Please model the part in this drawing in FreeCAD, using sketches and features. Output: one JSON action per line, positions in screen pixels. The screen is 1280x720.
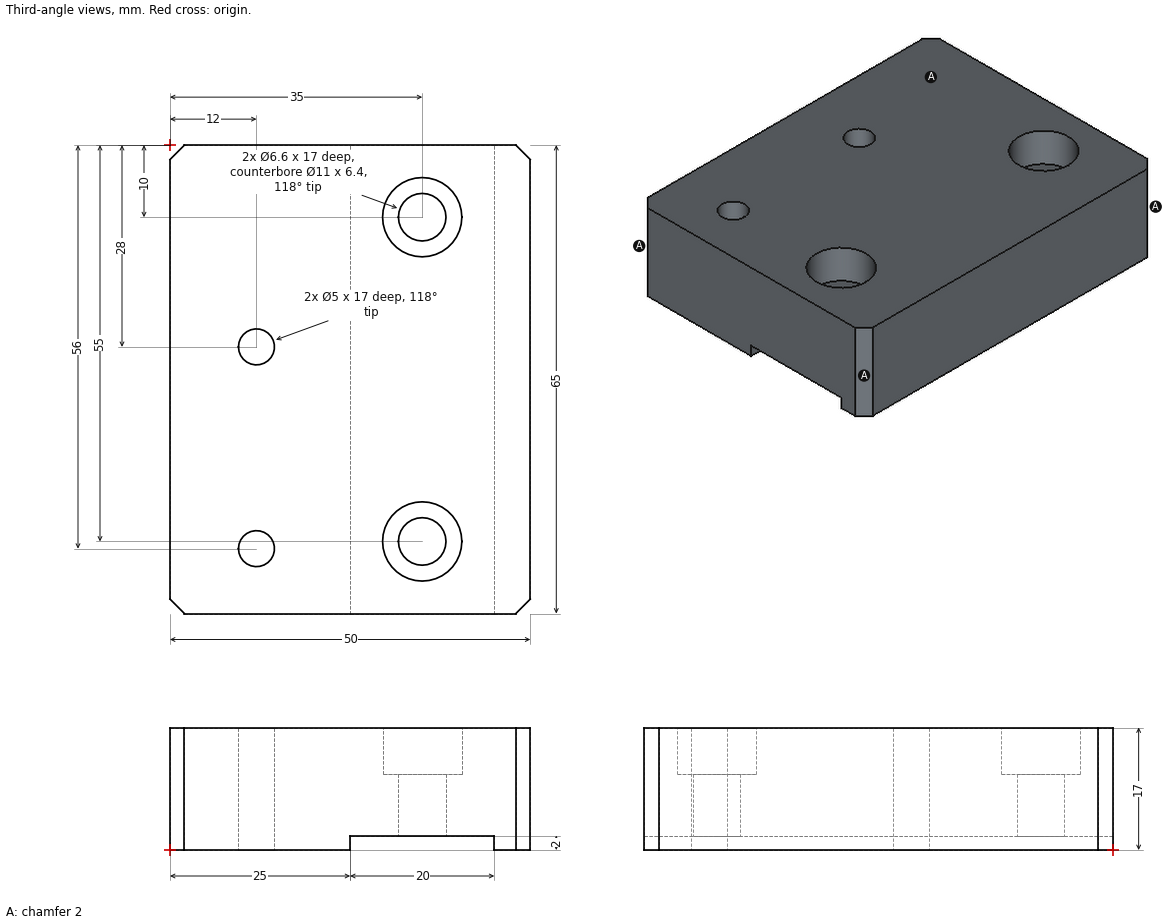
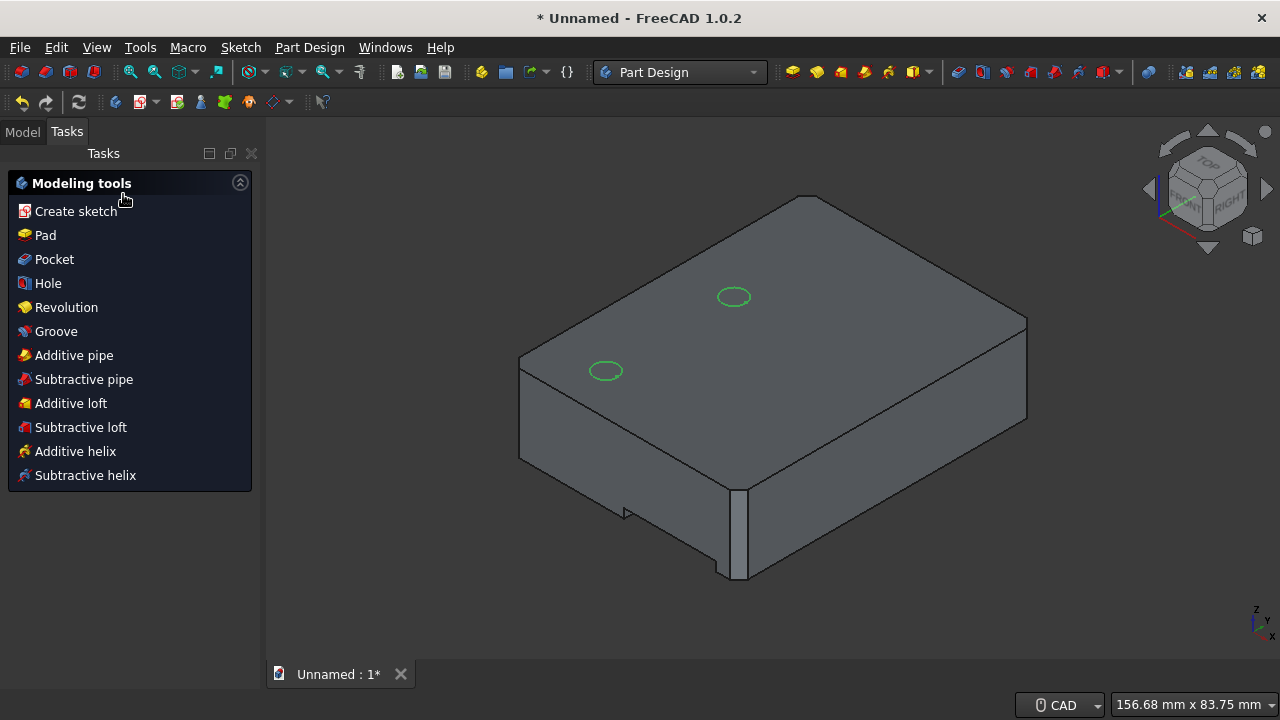
{"action": "left_click", "coordinate": [984, 72]}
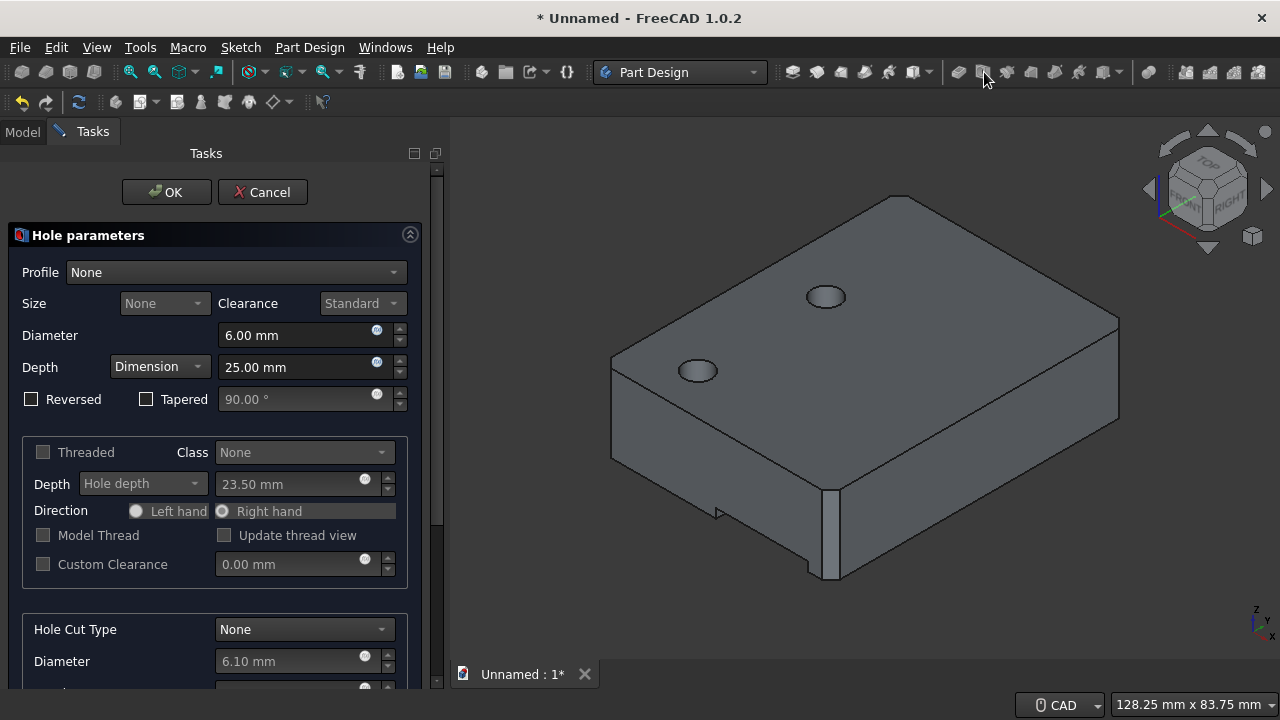
{"action": "triple_click", "coordinate": [305, 335]}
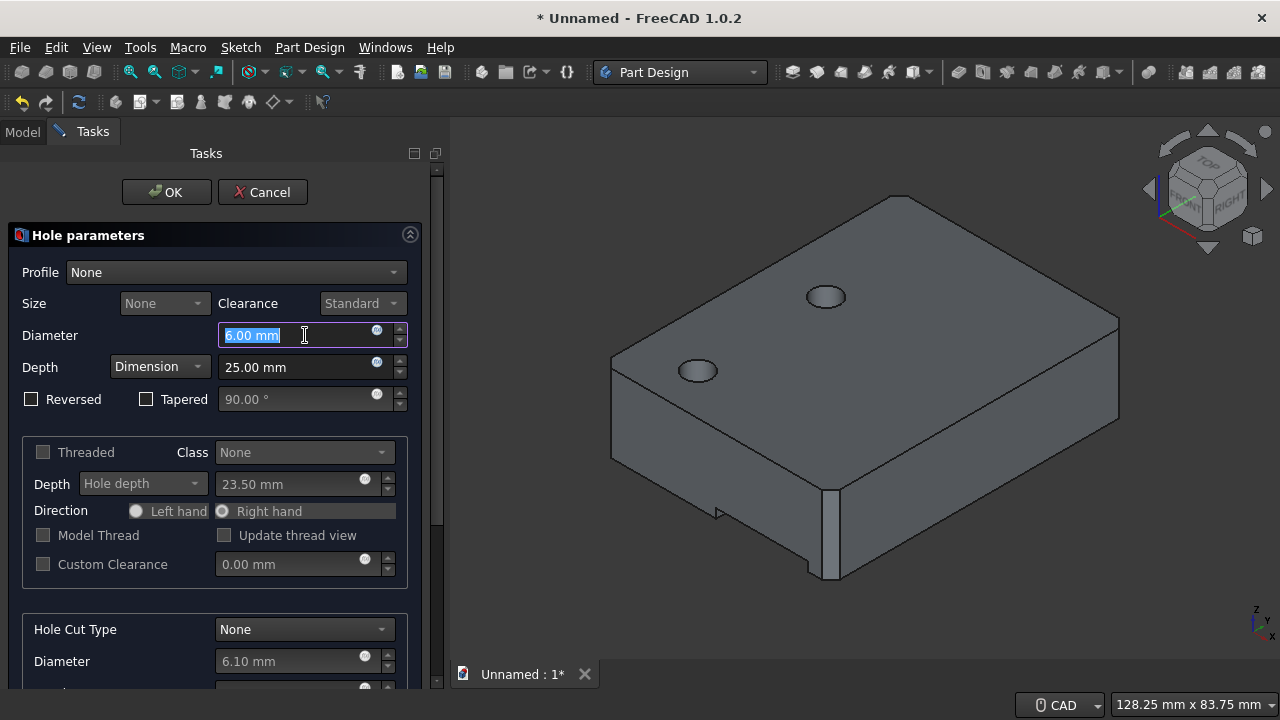
{"action": "type", "text": "5"}
{"action": "key", "text": "Tab"}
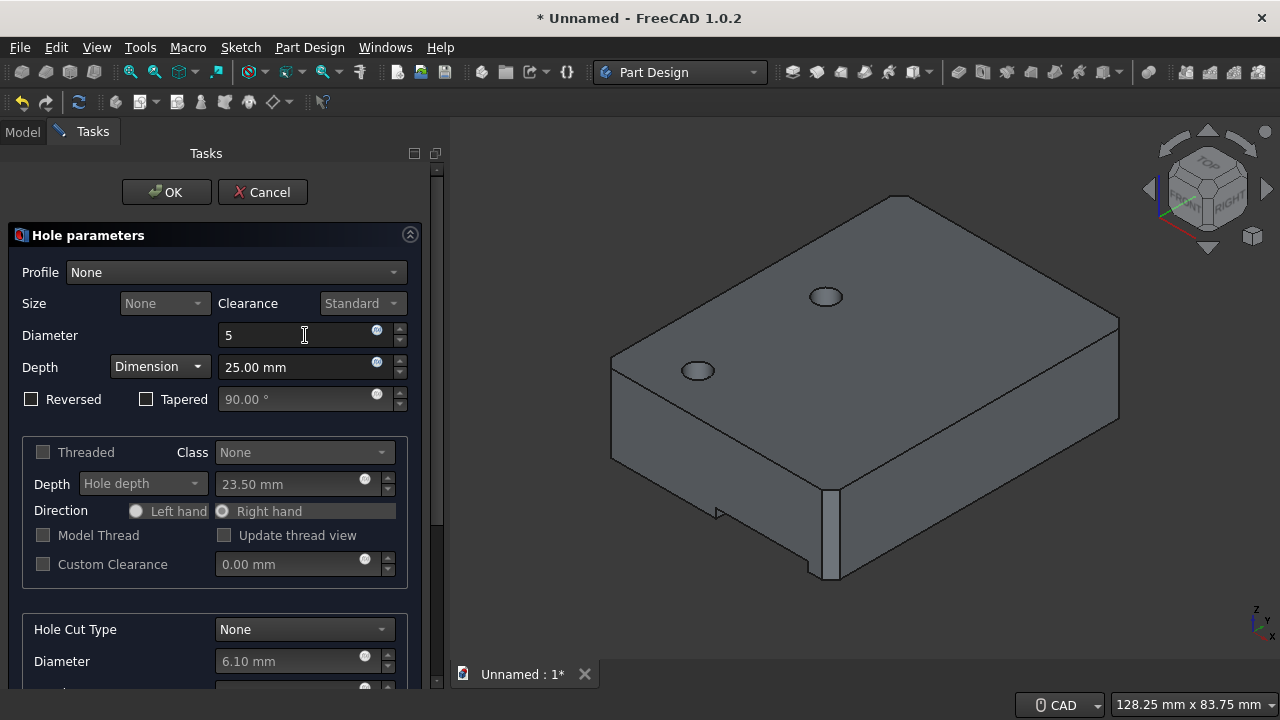
{"action": "triple_click", "coordinate": [305, 367]}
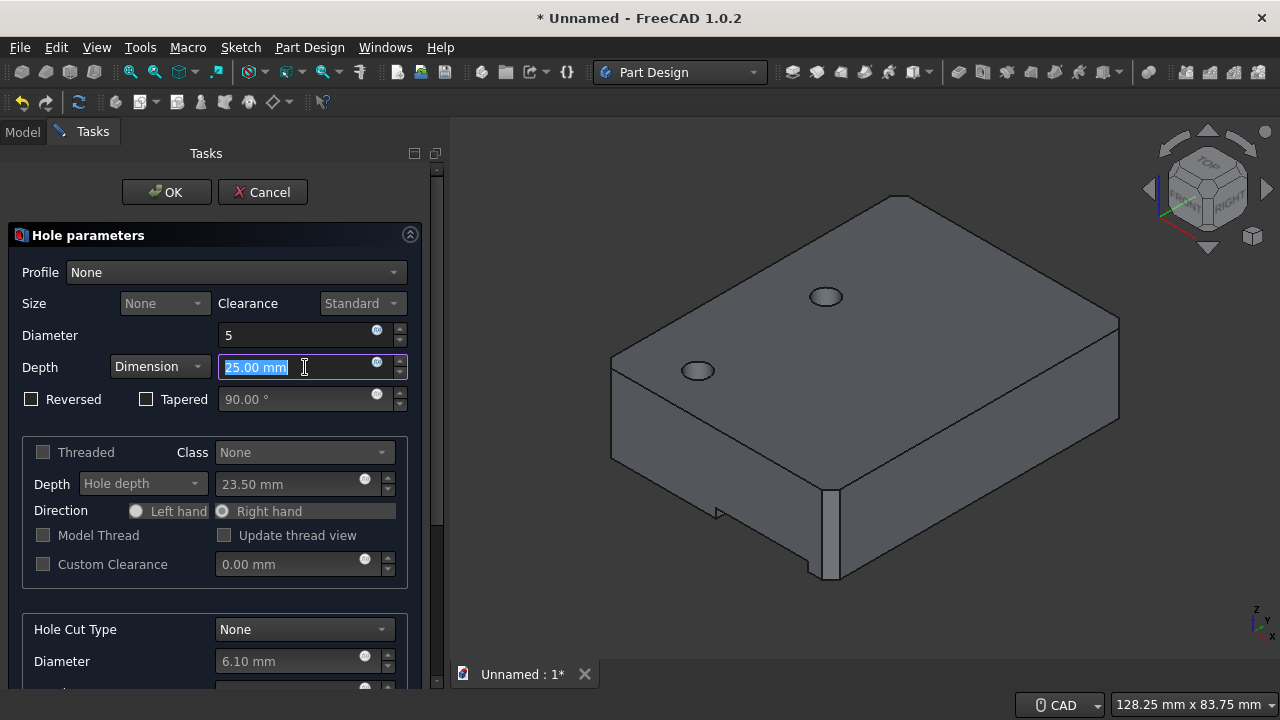
{"action": "type", "text": "17"}
{"action": "key", "text": "Tab"}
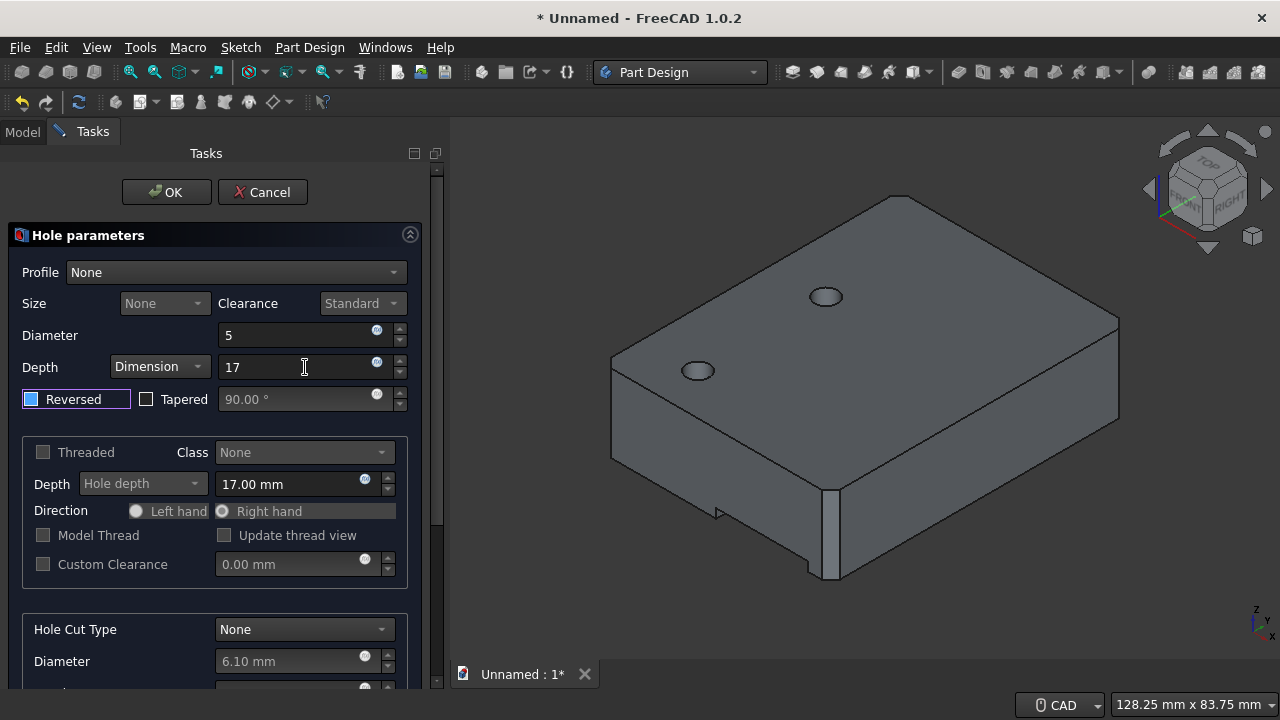
{"action": "left_click", "coordinate": [167, 192]}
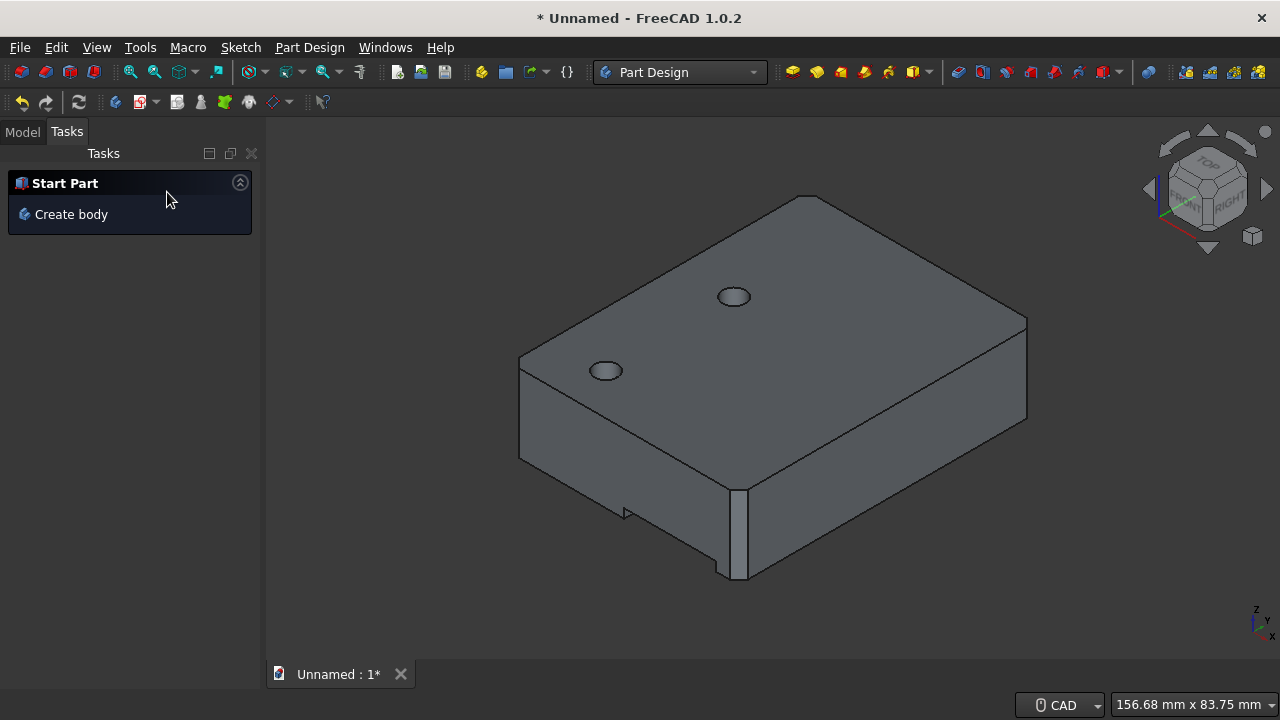
{"action": "left_click", "coordinate": [848, 336]}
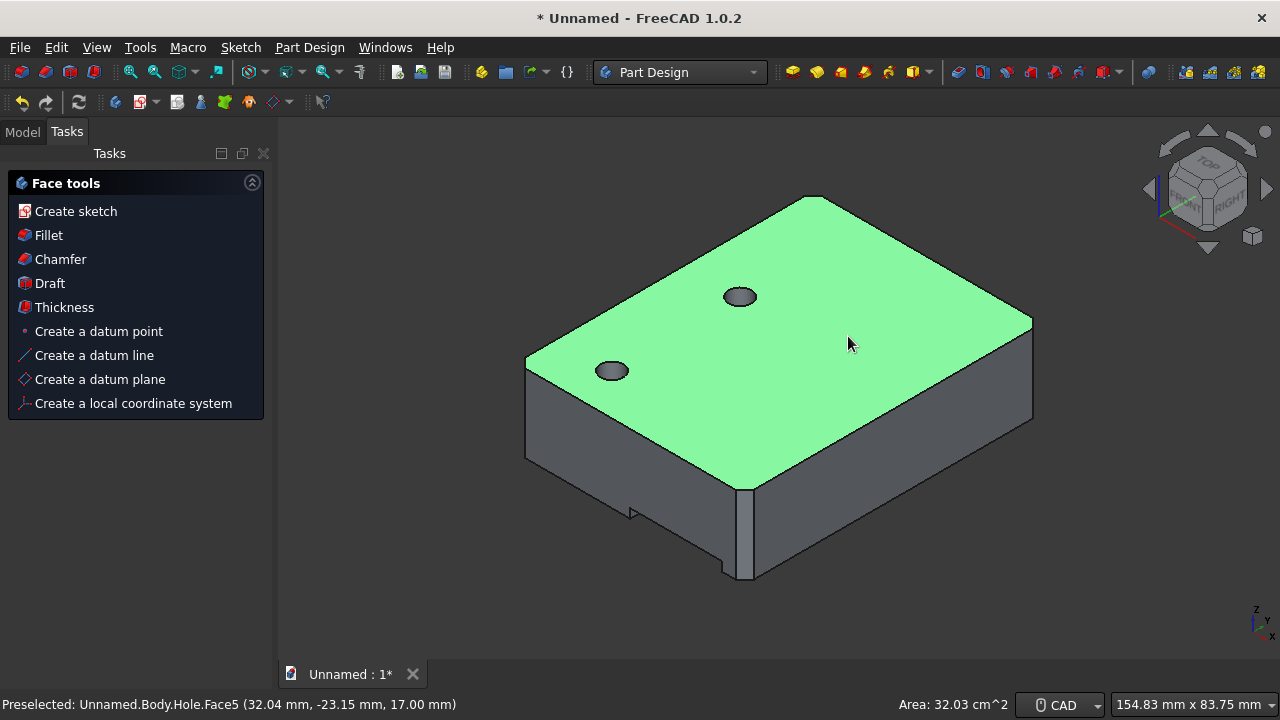
{"action": "left_click", "coordinate": [140, 102]}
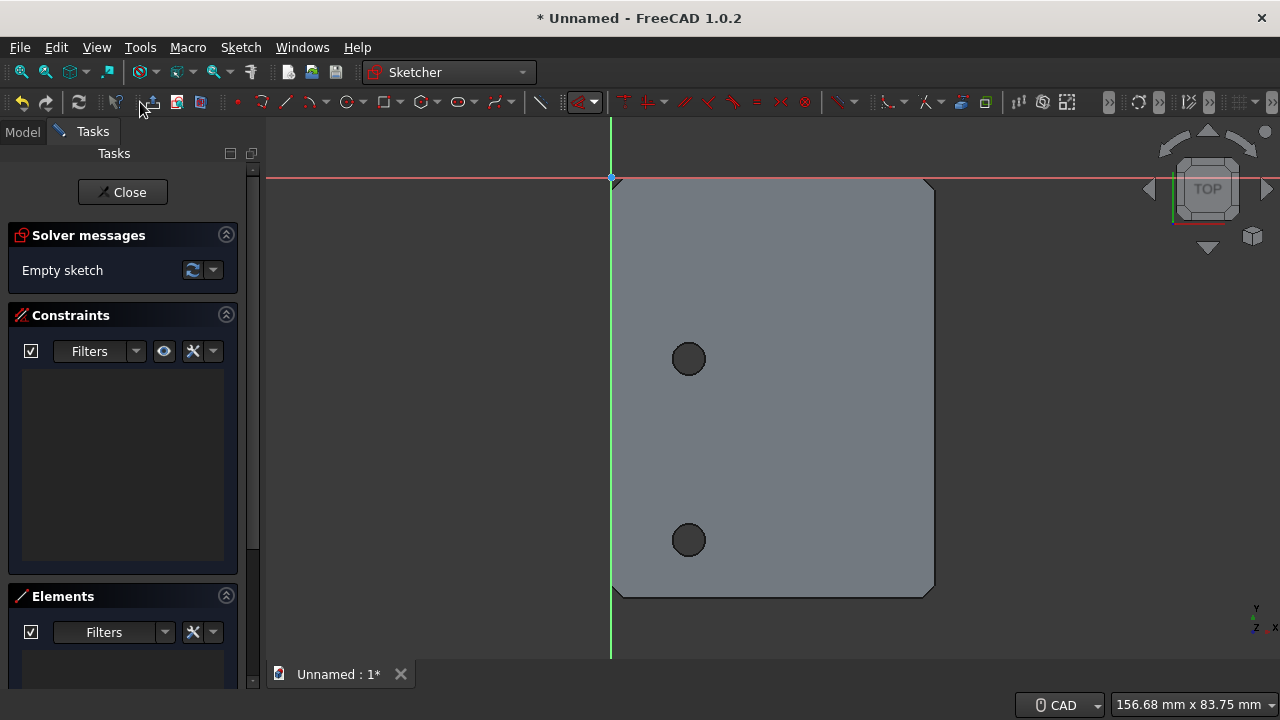
{"action": "left_click", "coordinate": [348, 102]}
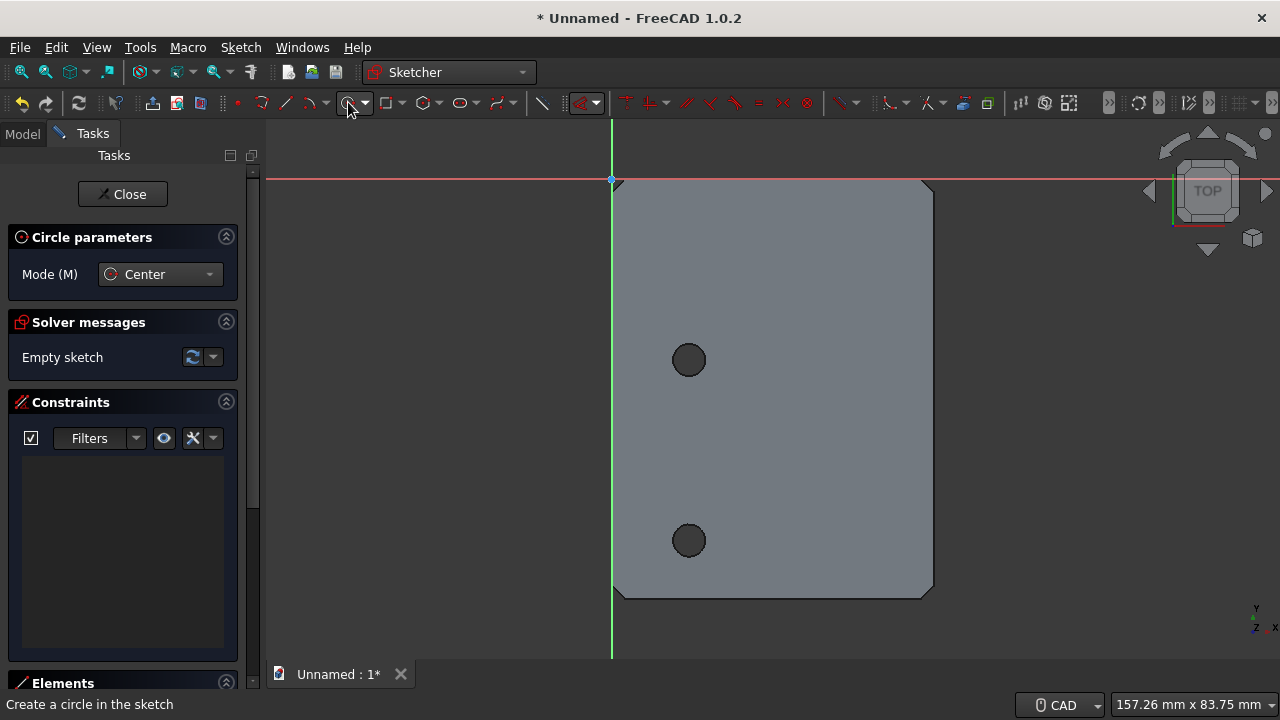
{"action": "left_click", "coordinate": [837, 244]}
{"action": "mouse_move", "coordinate": [853, 229]}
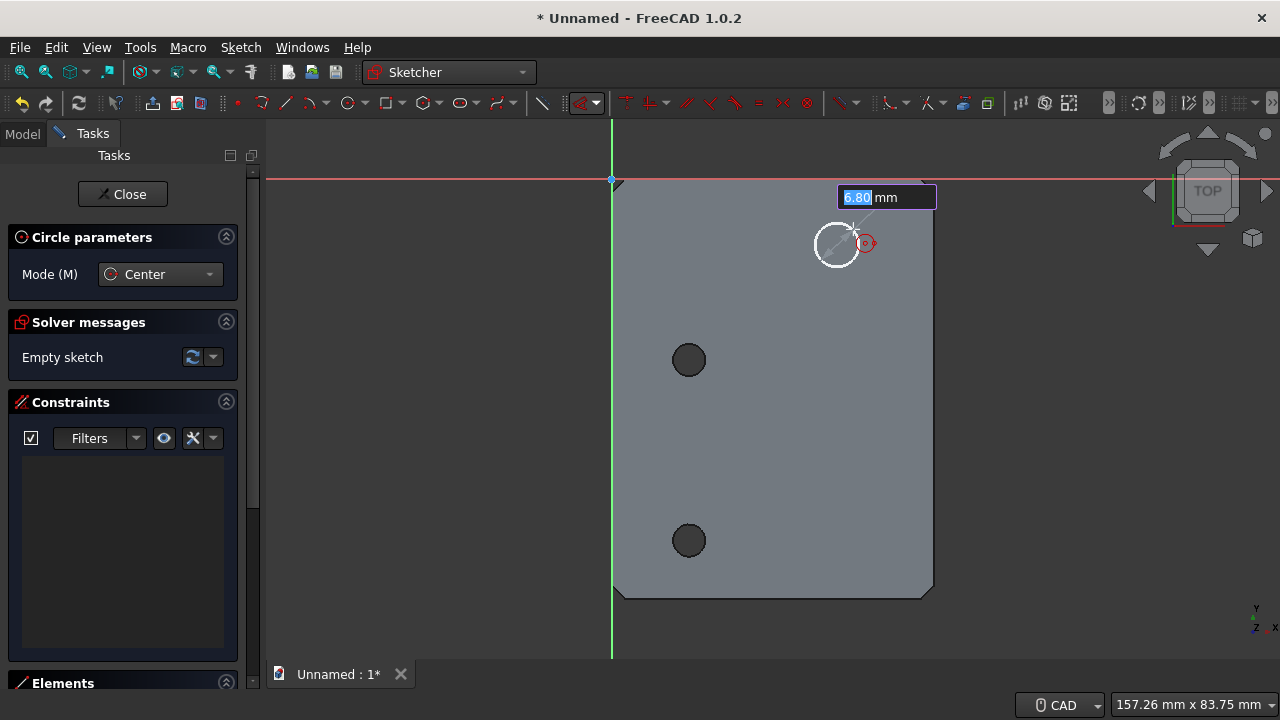
{"action": "type", "text": "6.6"}
{"action": "key", "text": "Return"}